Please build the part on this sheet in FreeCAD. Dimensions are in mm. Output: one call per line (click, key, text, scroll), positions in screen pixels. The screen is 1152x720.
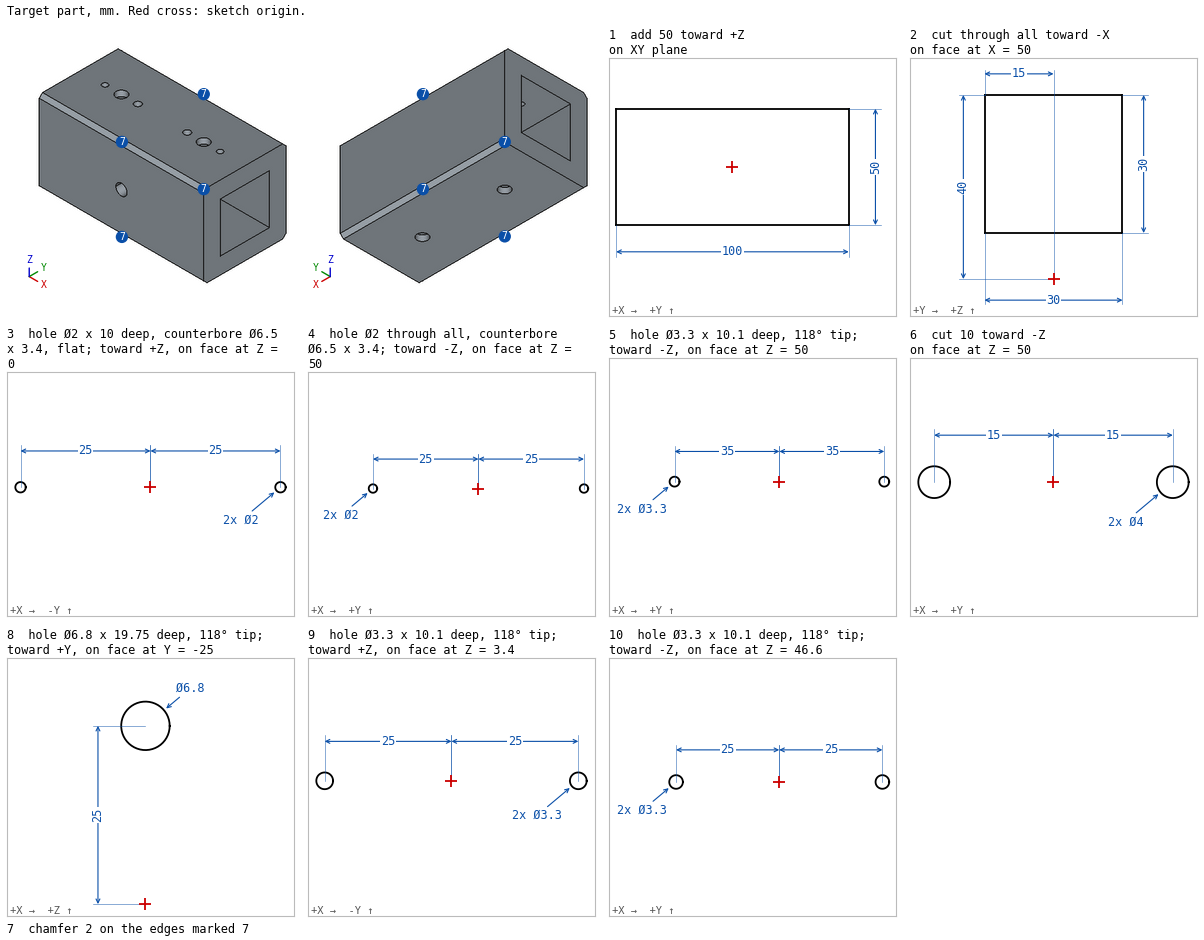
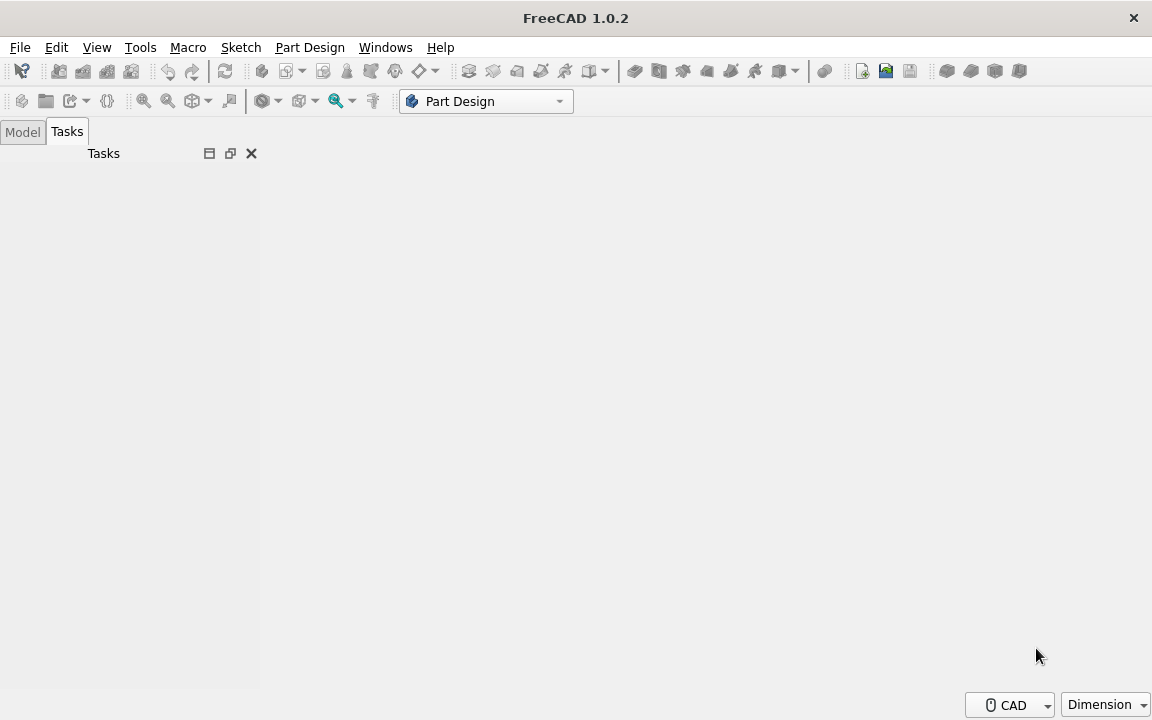
click(862, 72)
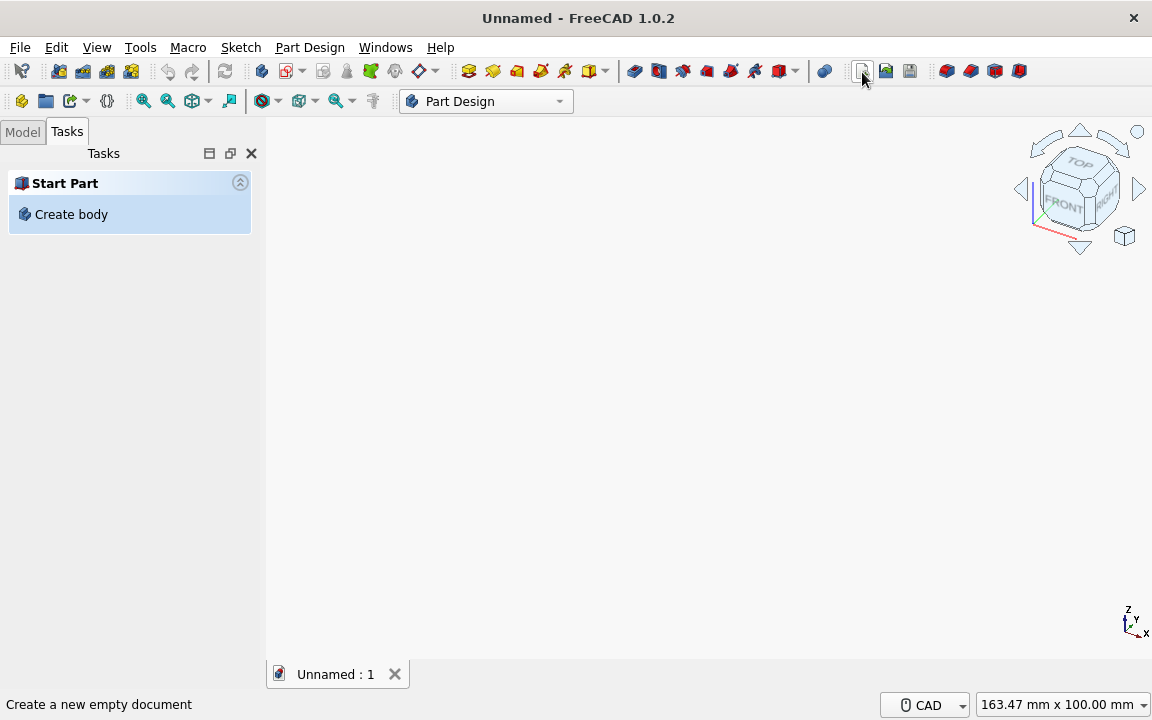
click(286, 72)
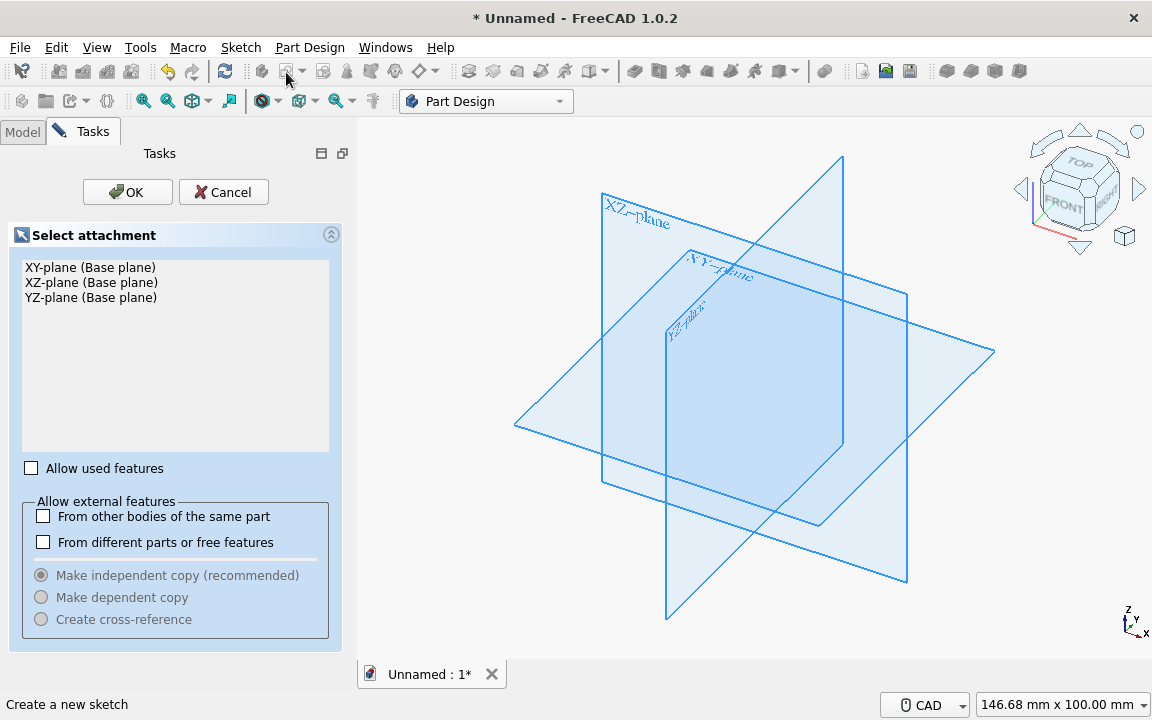
click(82, 268)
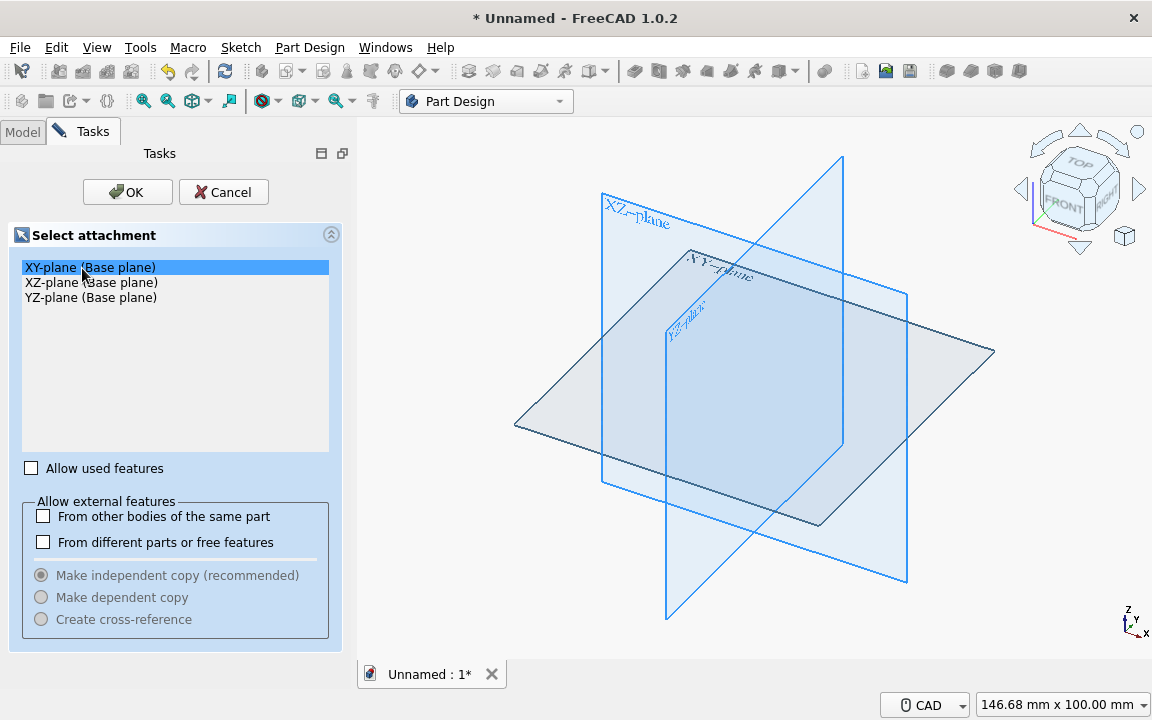
click(128, 192)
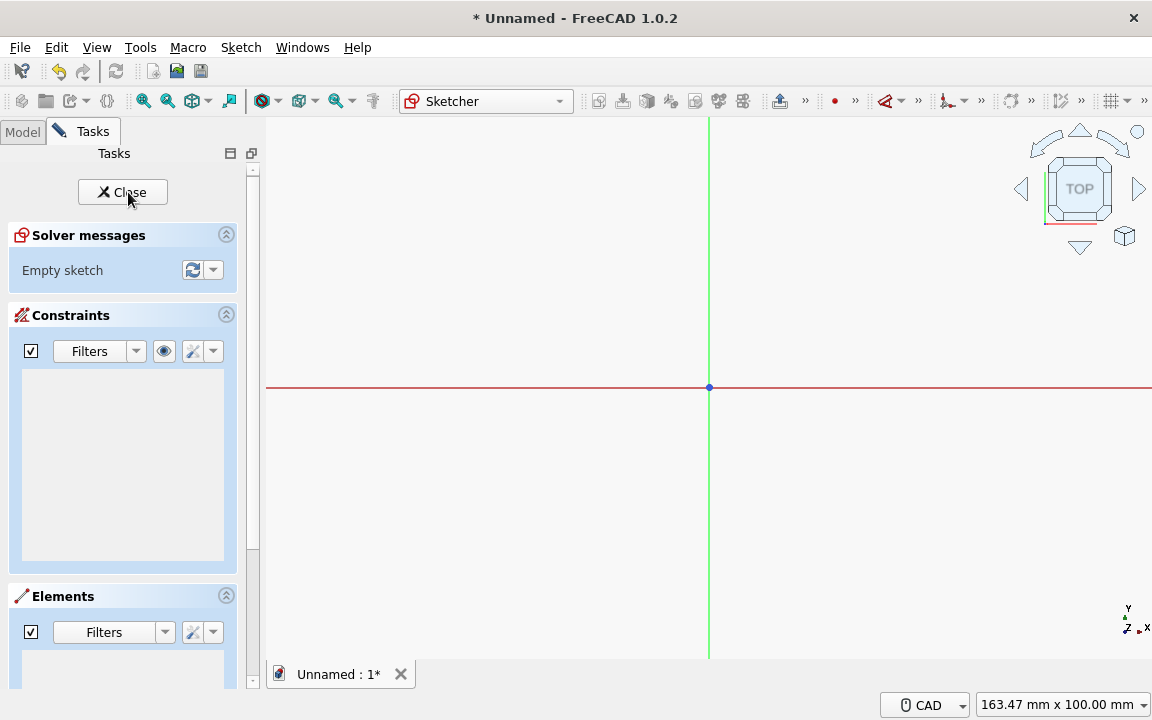
scroll(331, 388, down, 1)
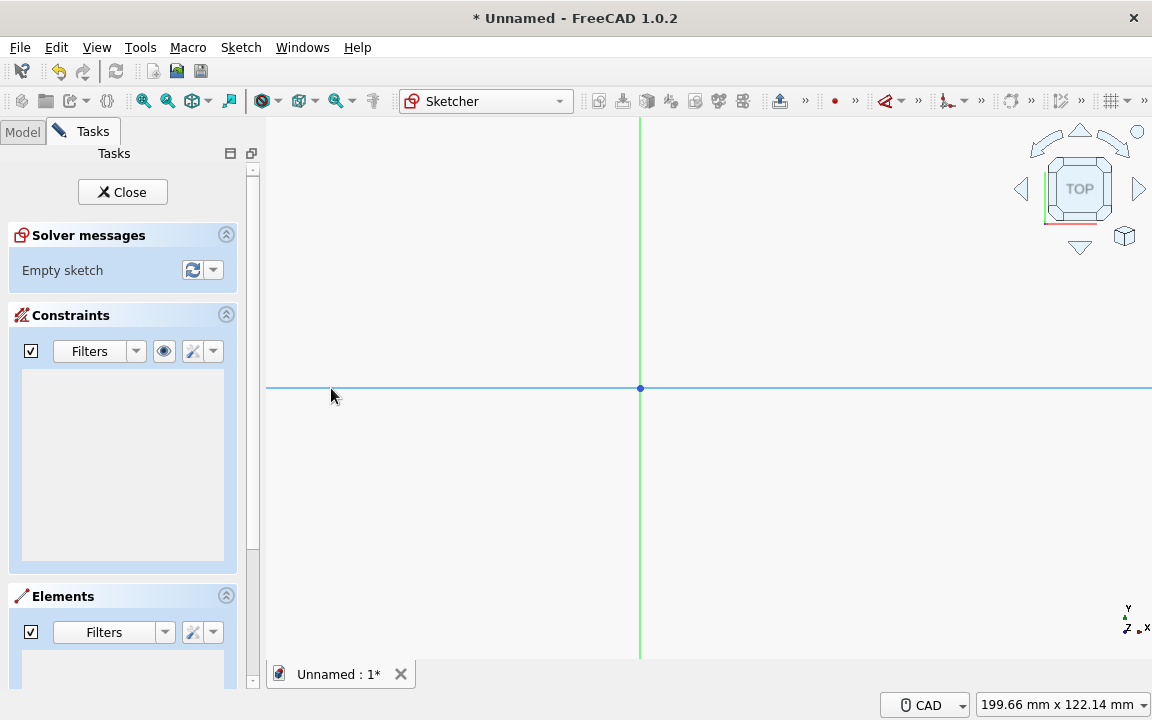
key(g)
key(v)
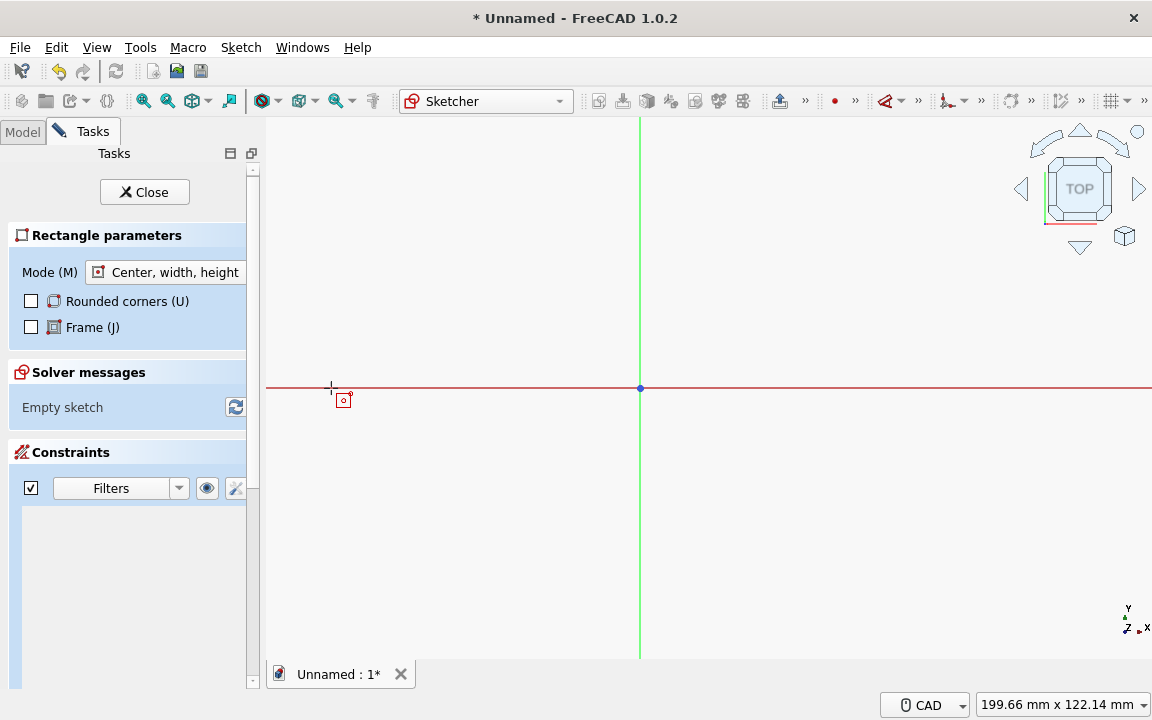
click(640, 388)
move(862, 277)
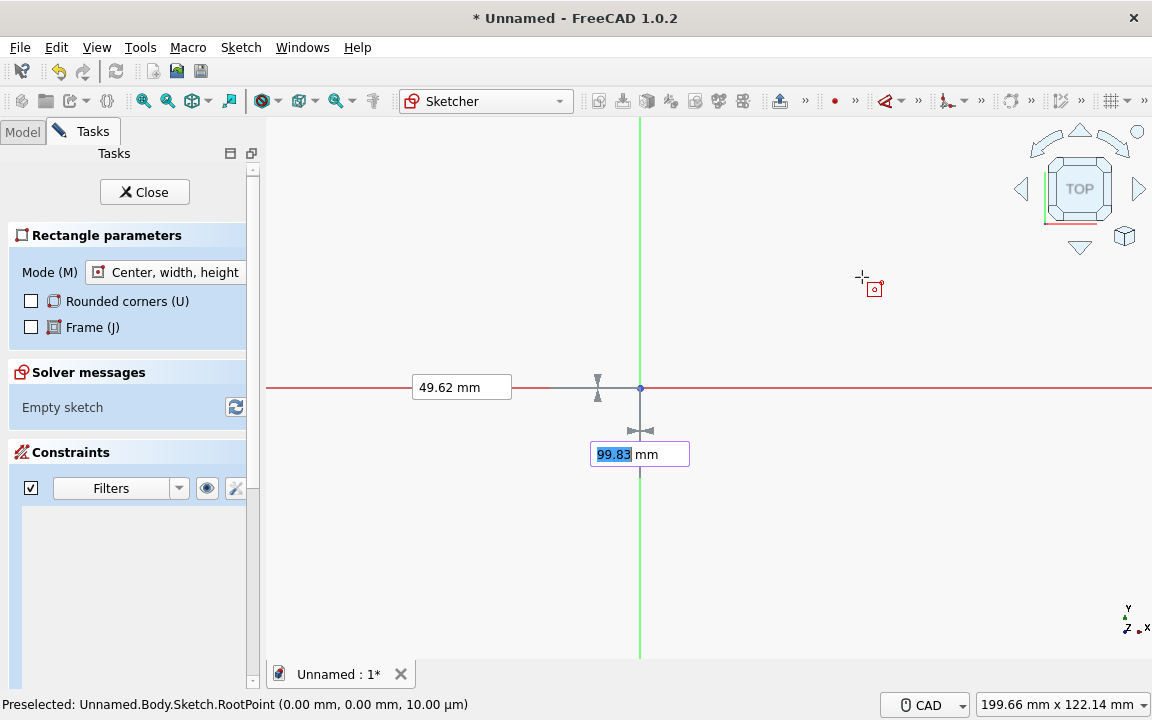
text(100)
key(Tab)
text(50)
key(Return)
key(Escape)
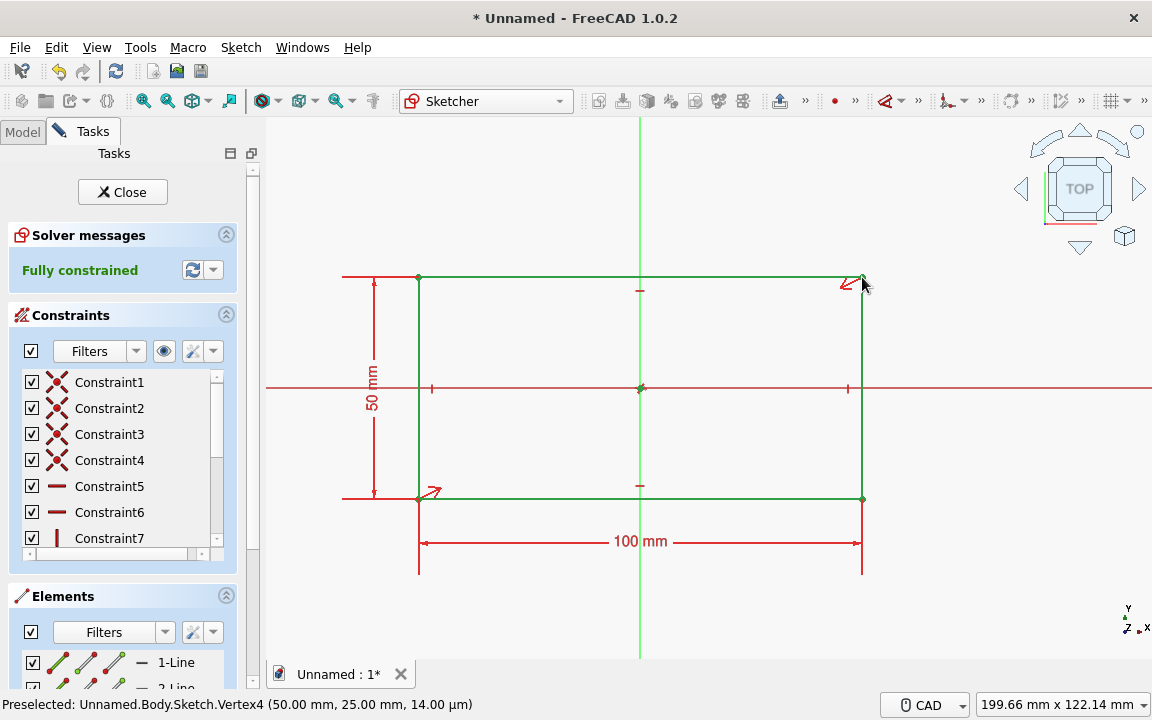
click(123, 192)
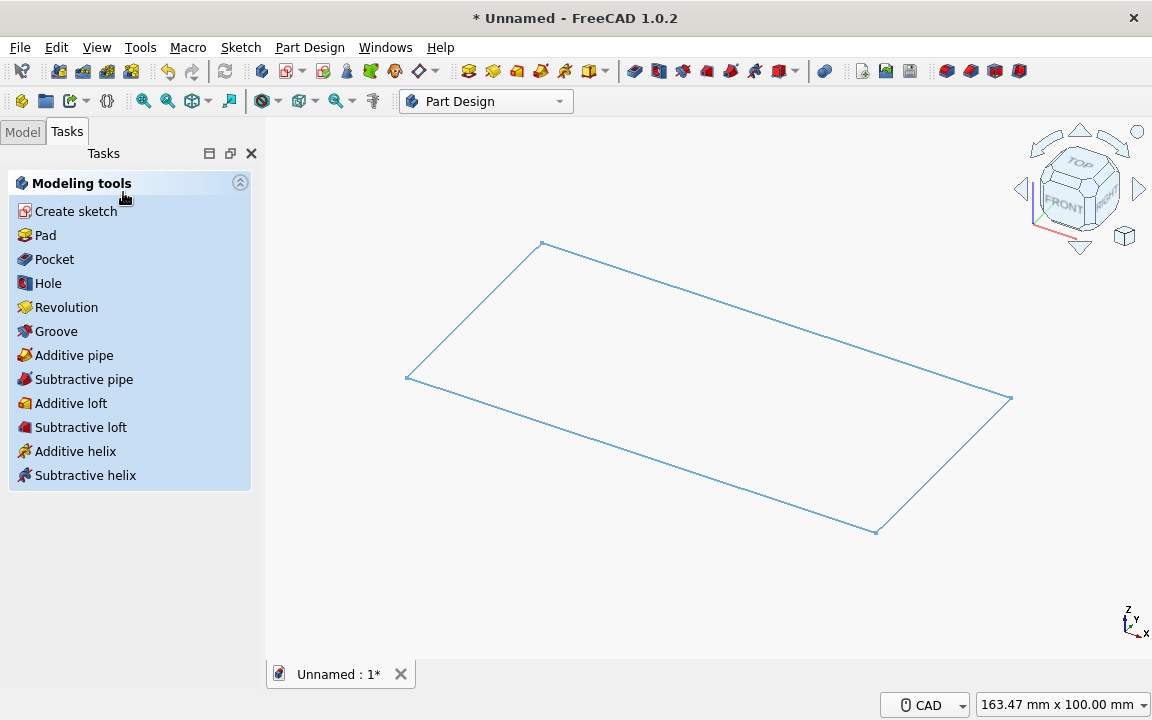
click(470, 72)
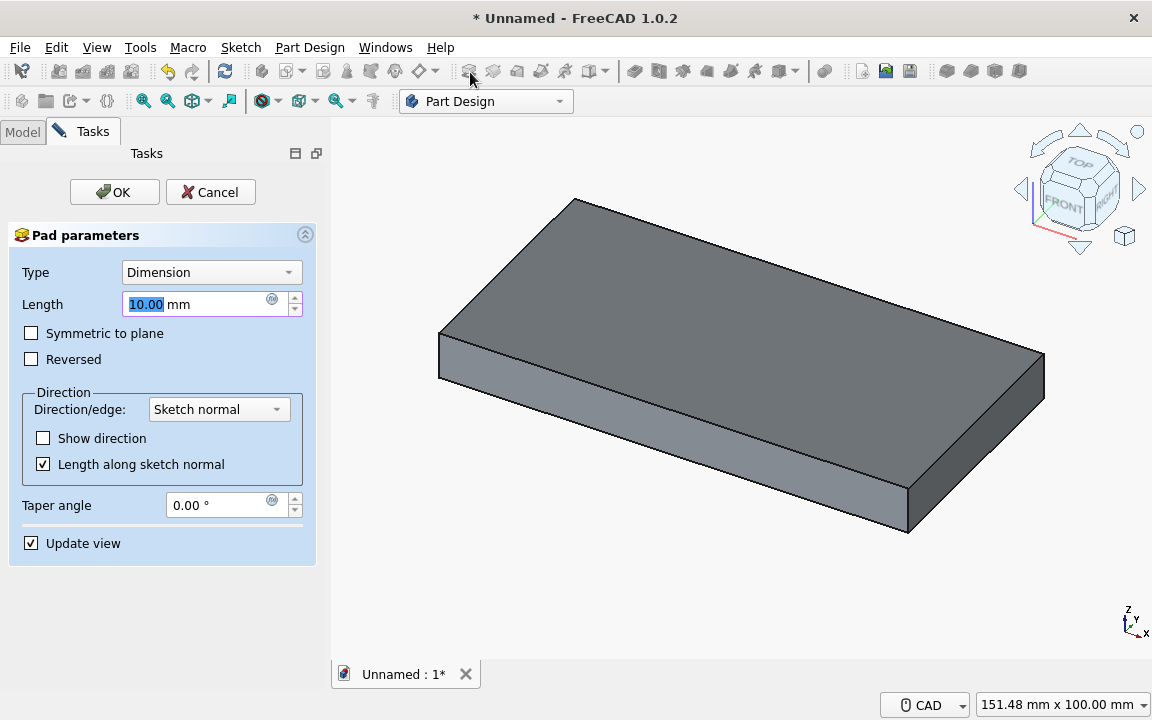
text(50)
key(Tab)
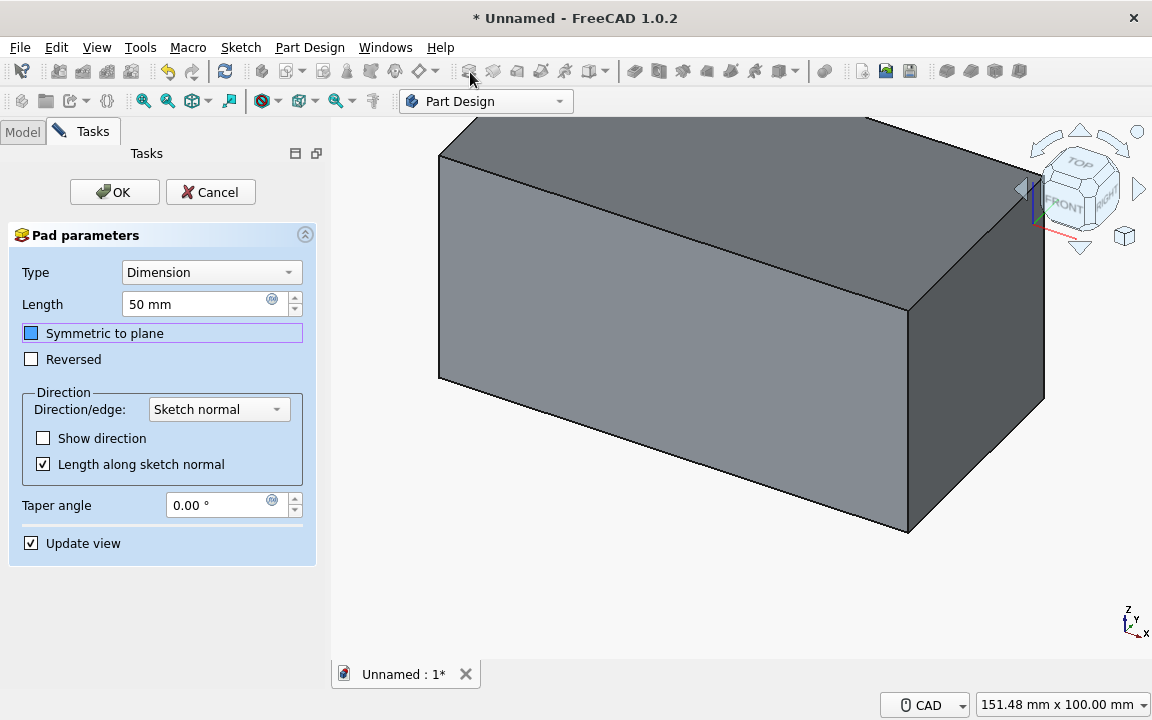
click(115, 192)